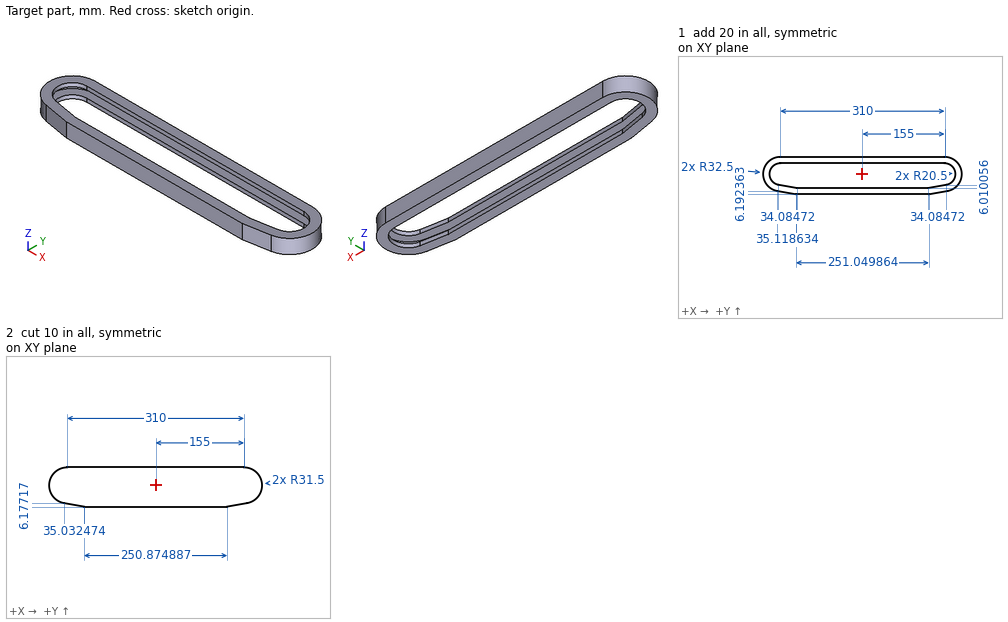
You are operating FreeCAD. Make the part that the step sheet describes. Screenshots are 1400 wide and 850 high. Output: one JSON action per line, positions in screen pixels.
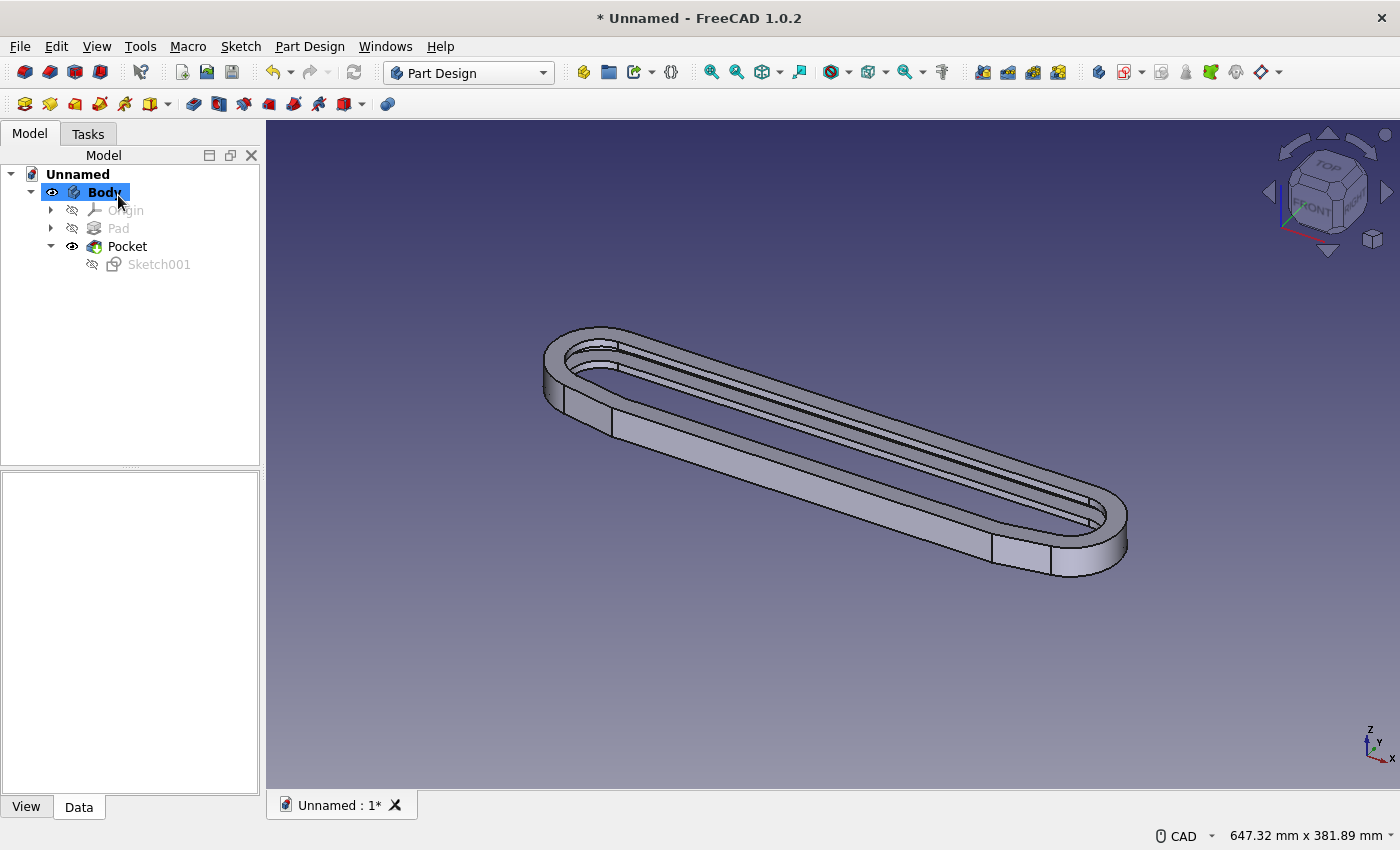
{"action": "key", "text": "0"}